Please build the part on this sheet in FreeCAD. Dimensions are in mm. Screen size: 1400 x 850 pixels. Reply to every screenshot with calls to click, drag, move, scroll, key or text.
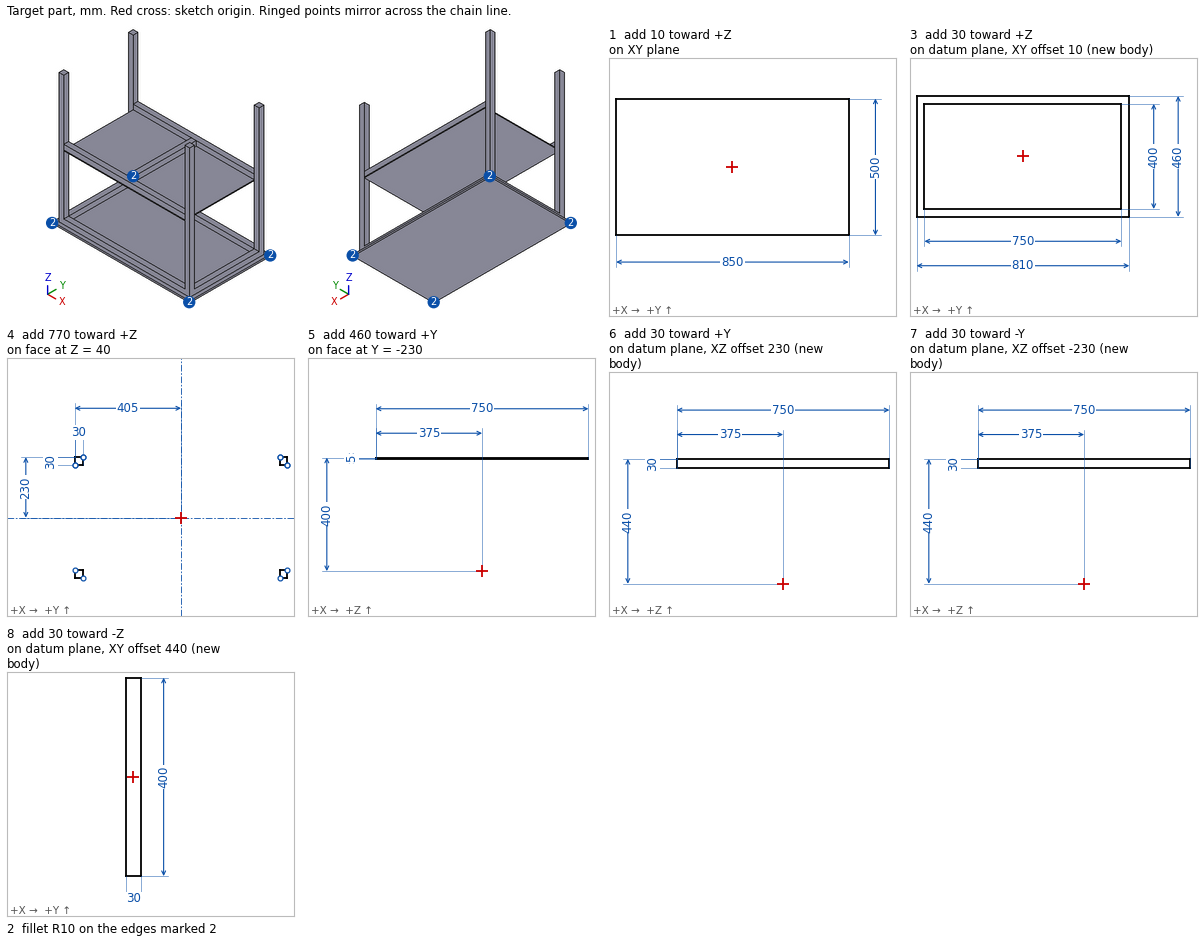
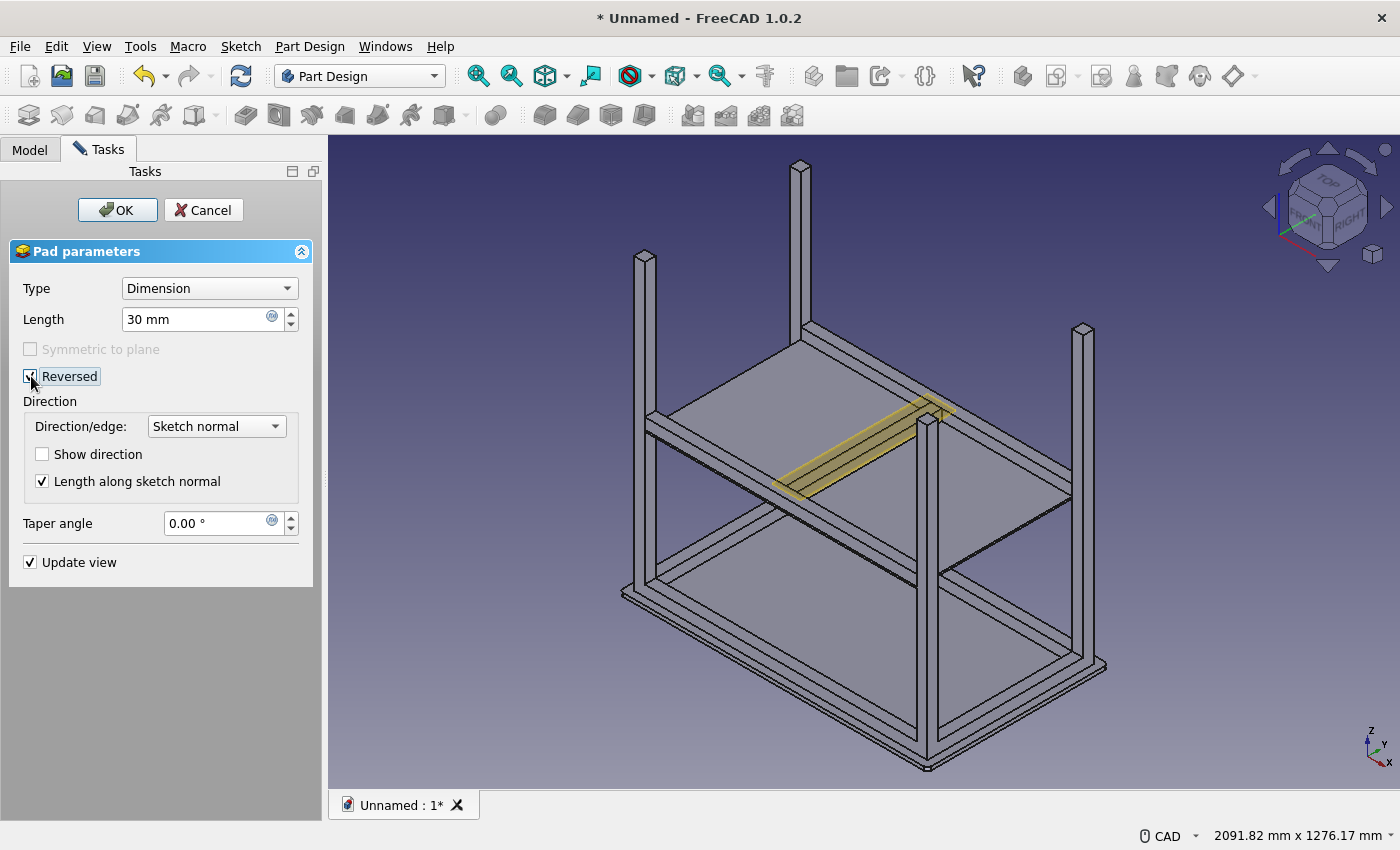
click(118, 210)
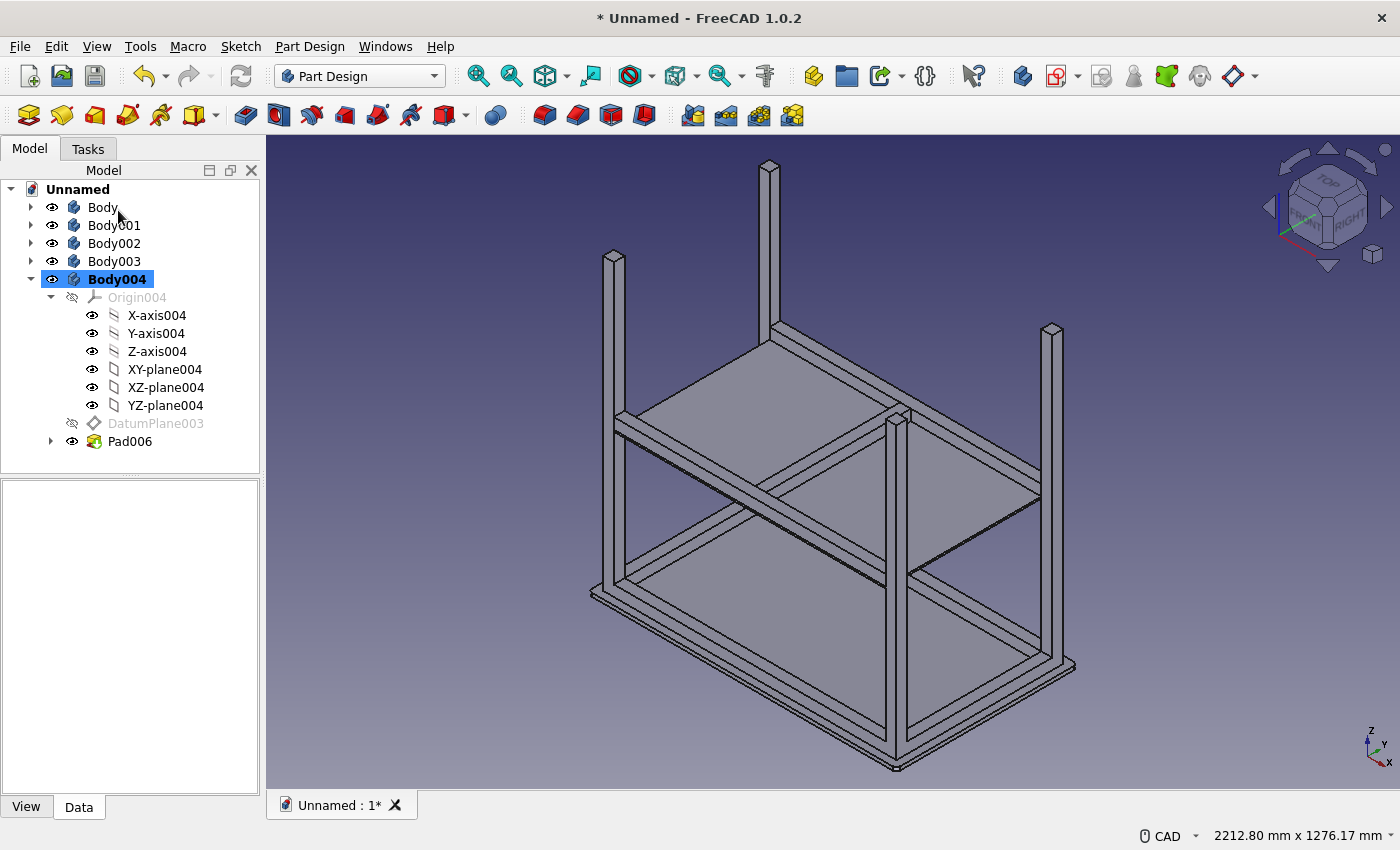
key(v)
key(f)